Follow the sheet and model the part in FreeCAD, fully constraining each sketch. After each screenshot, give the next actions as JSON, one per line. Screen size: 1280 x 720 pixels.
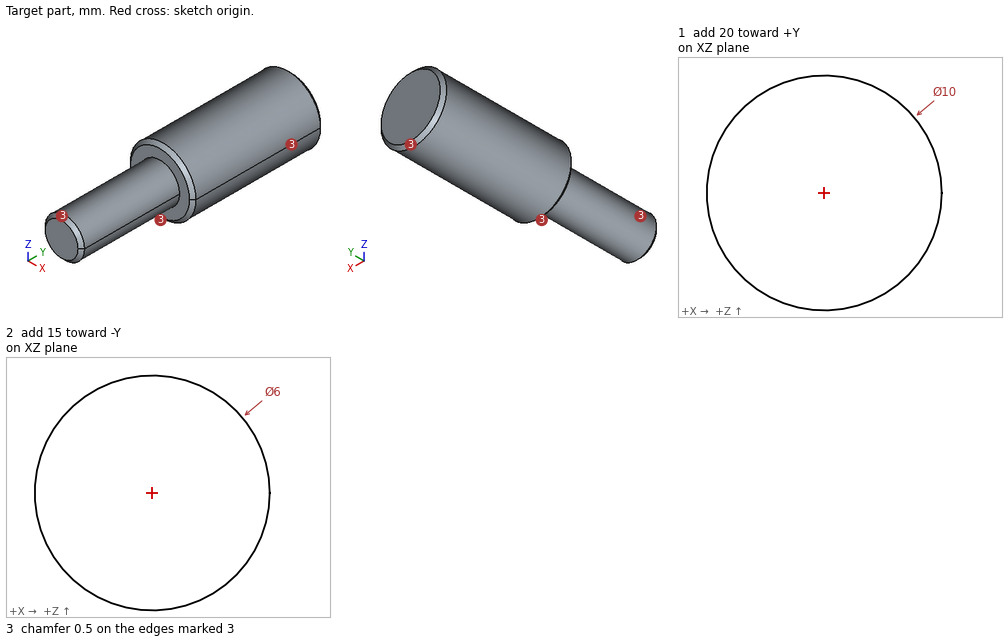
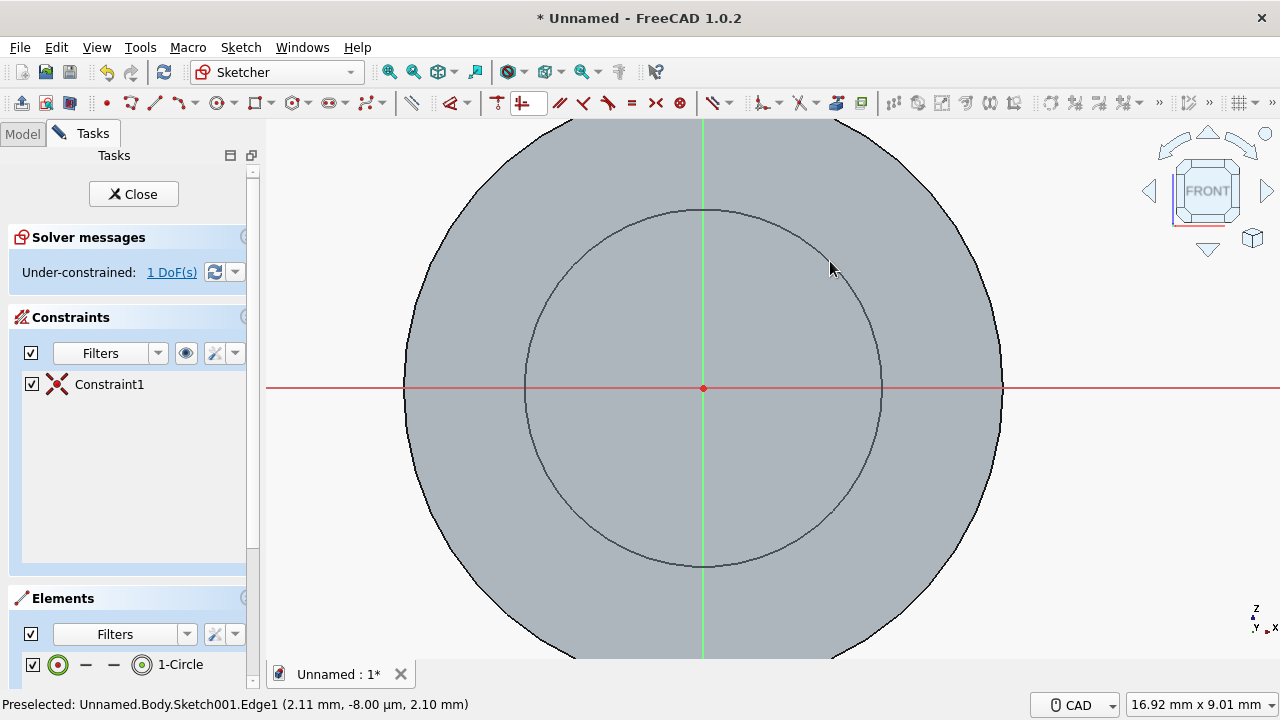
{"action": "left_click", "coordinate": [450, 104]}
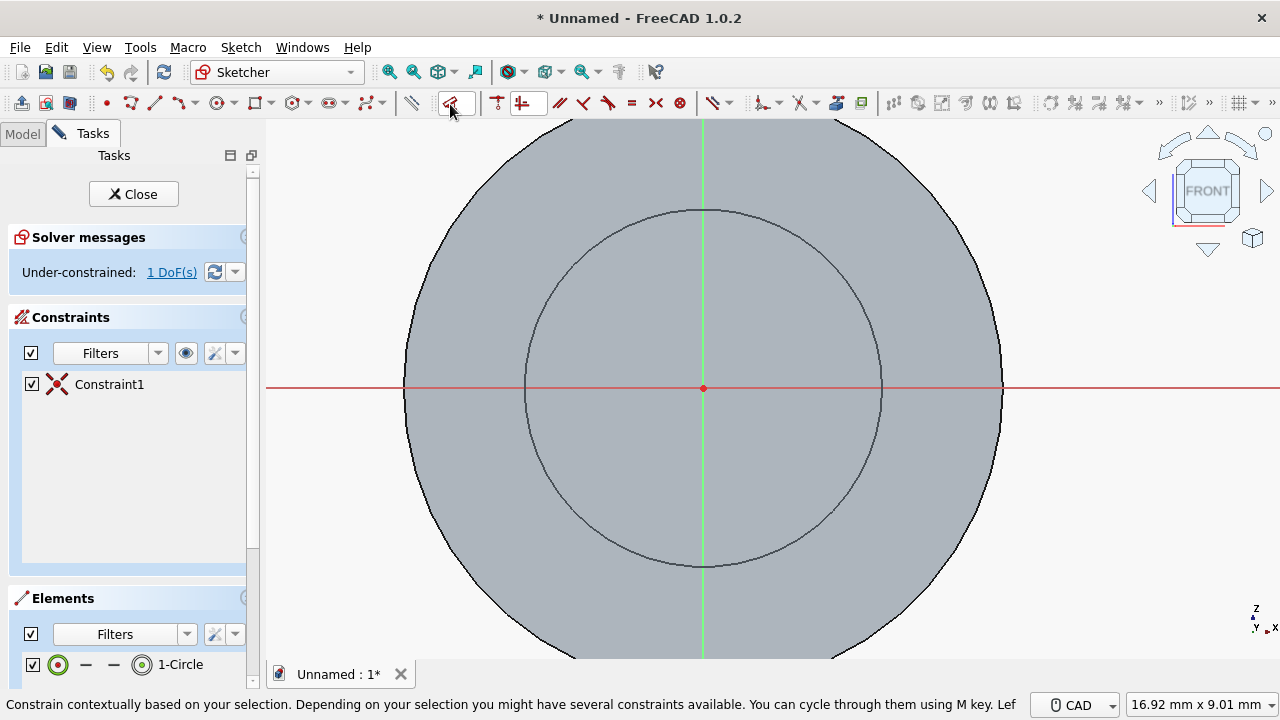
{"action": "left_click", "coordinate": [829, 261]}
{"action": "left_click", "coordinate": [851, 238]}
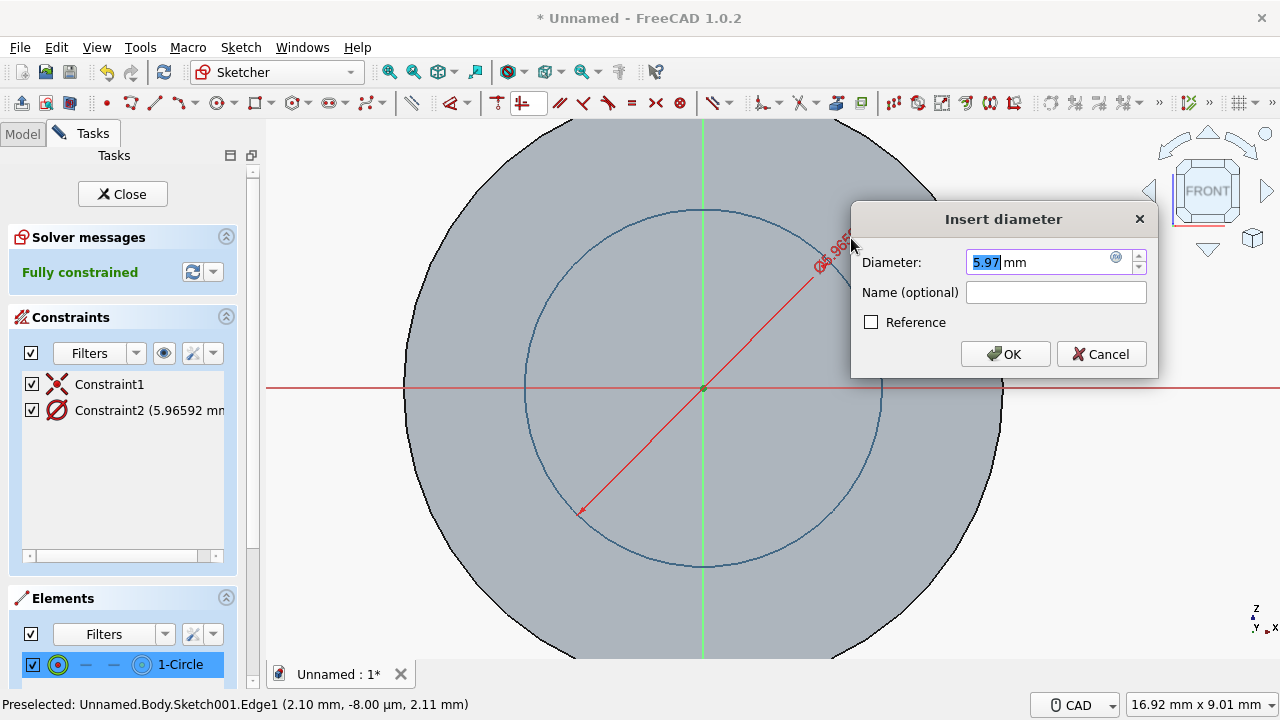
{"action": "type", "text": "6"}
{"action": "key", "text": "Return"}
{"action": "key", "text": "Escape"}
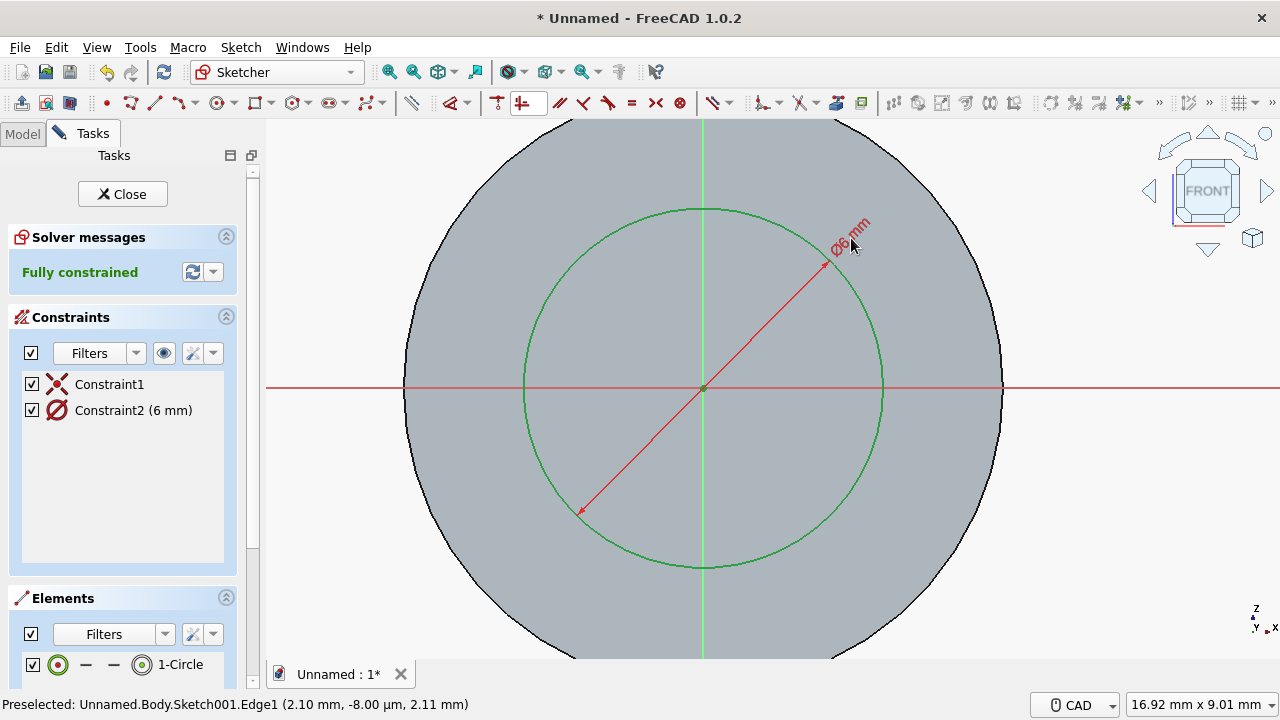
{"action": "left_click", "coordinate": [123, 194]}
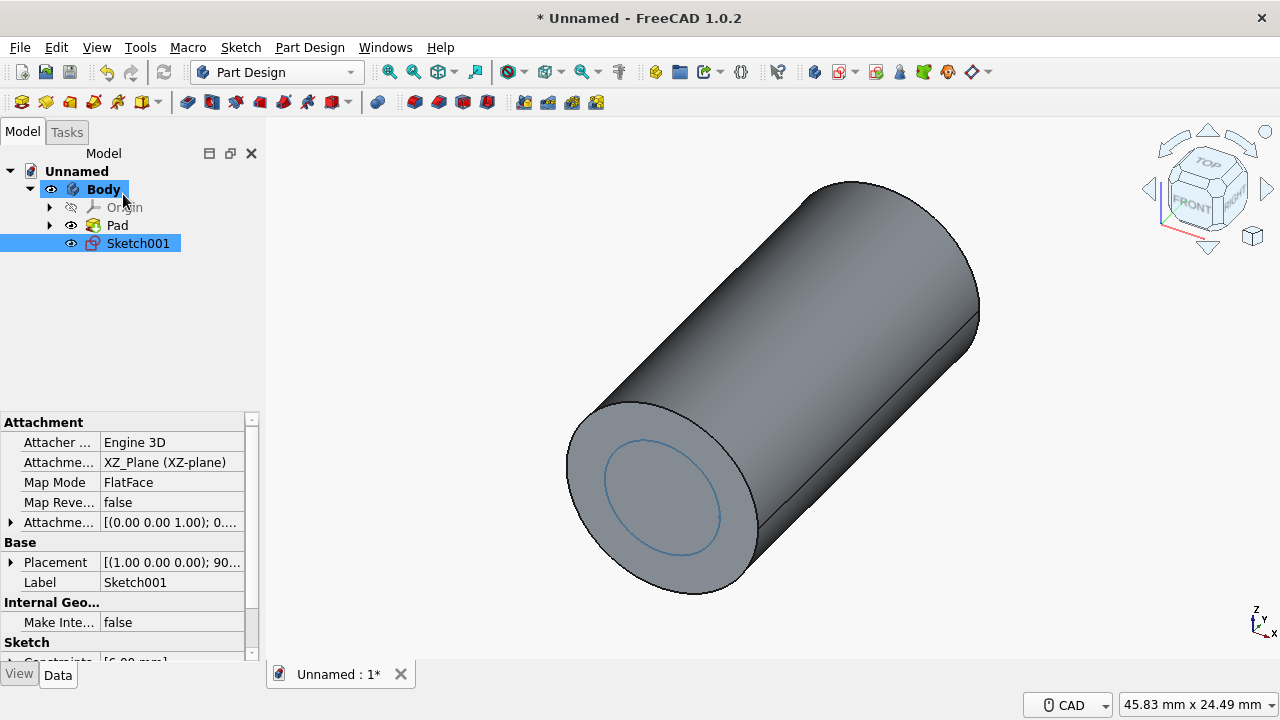
{"action": "left_click", "coordinate": [22, 102]}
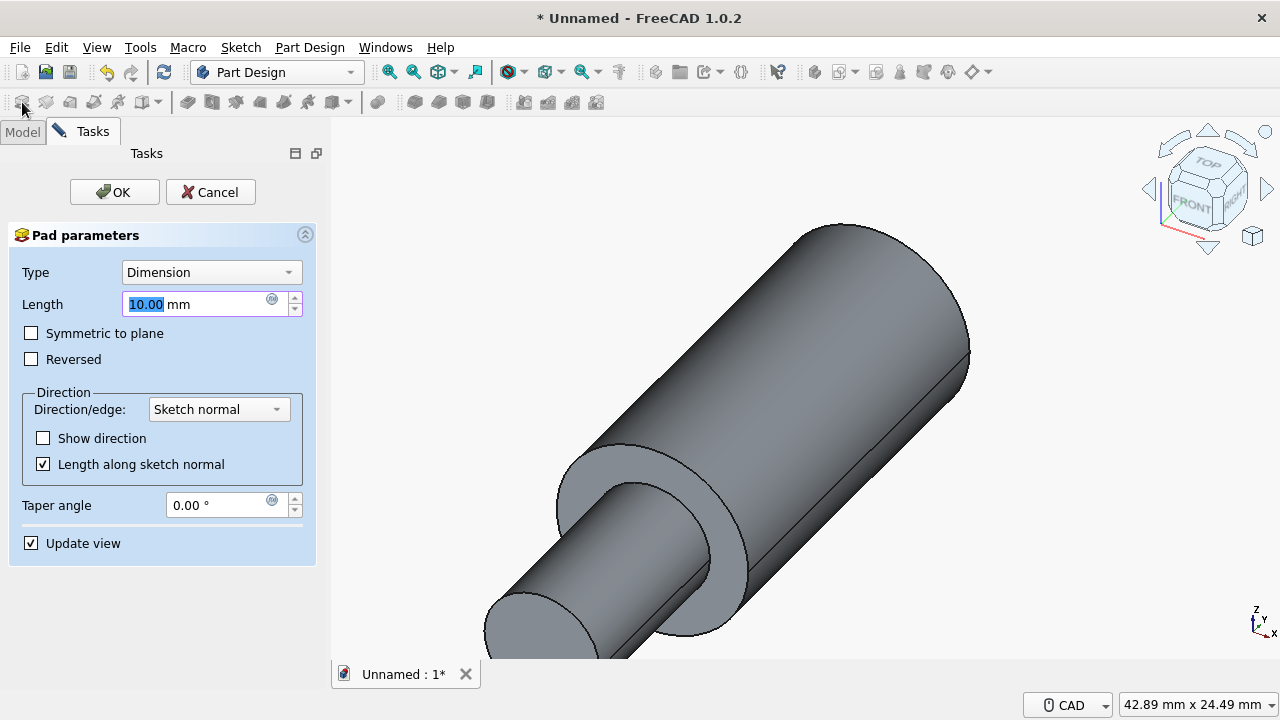
{"action": "type", "text": "15"}
{"action": "key", "text": "Tab"}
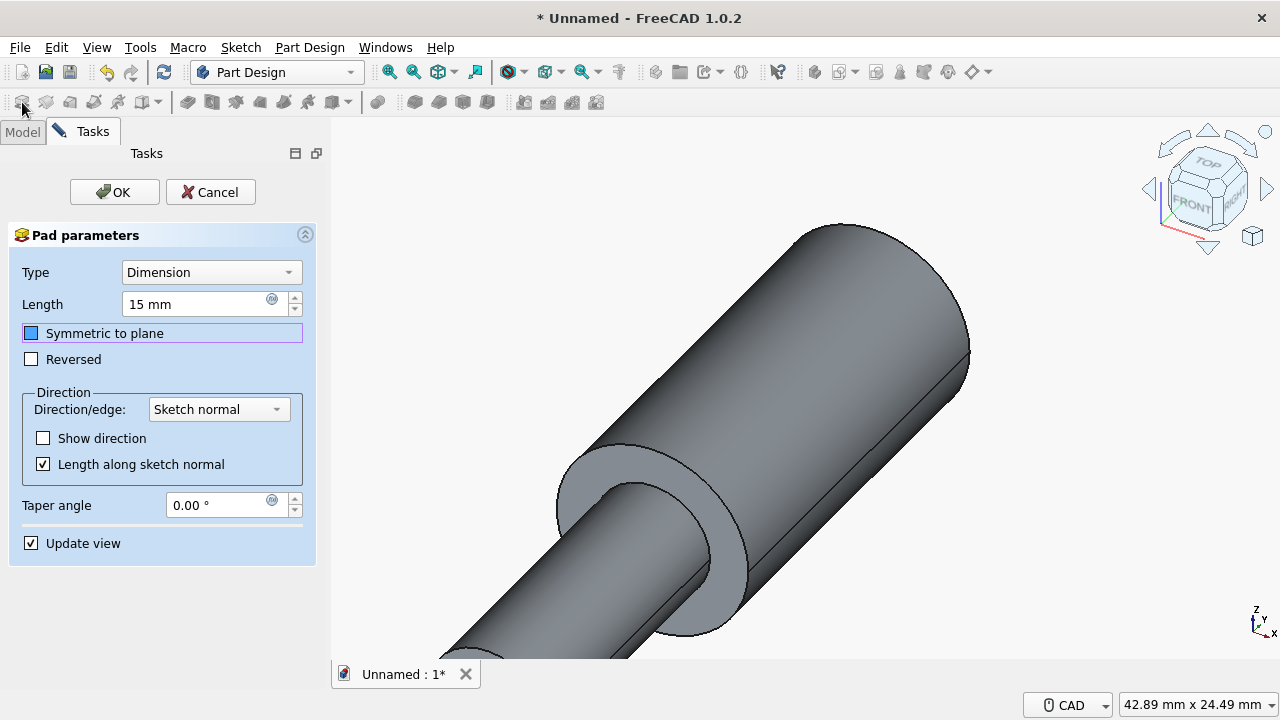
{"action": "left_click", "coordinate": [115, 192]}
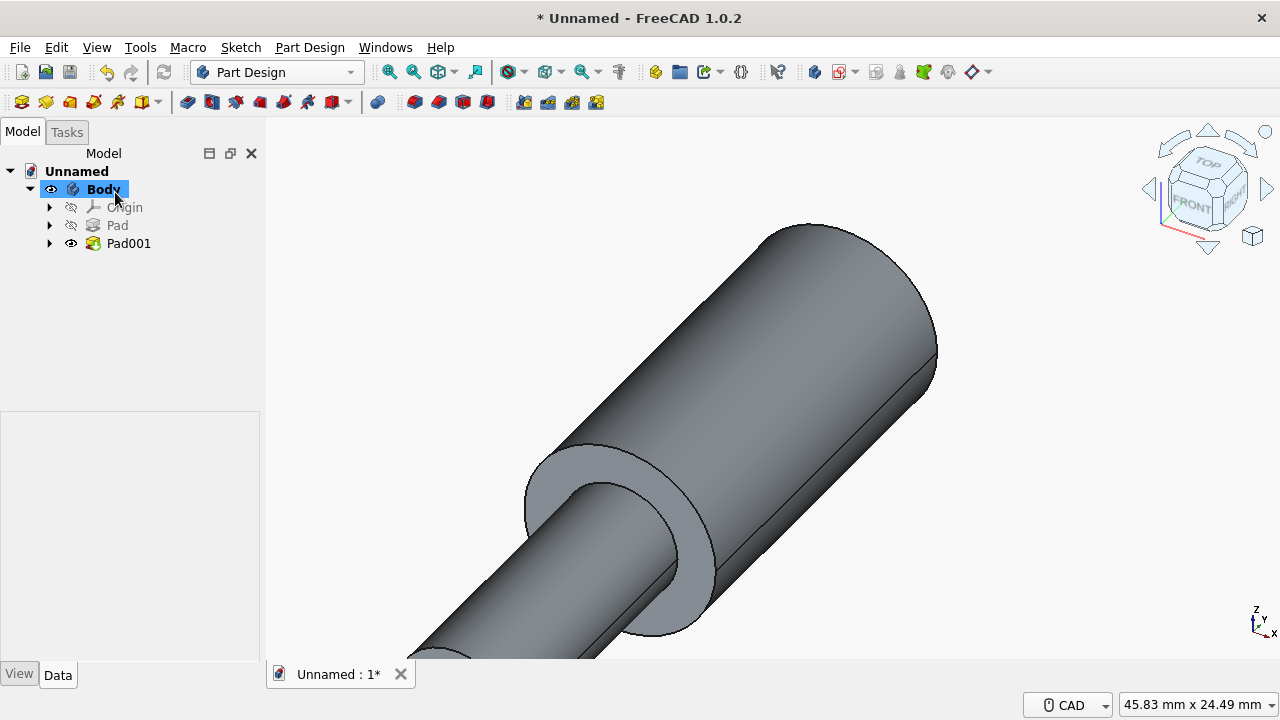
{"action": "left_click", "coordinate": [390, 72]}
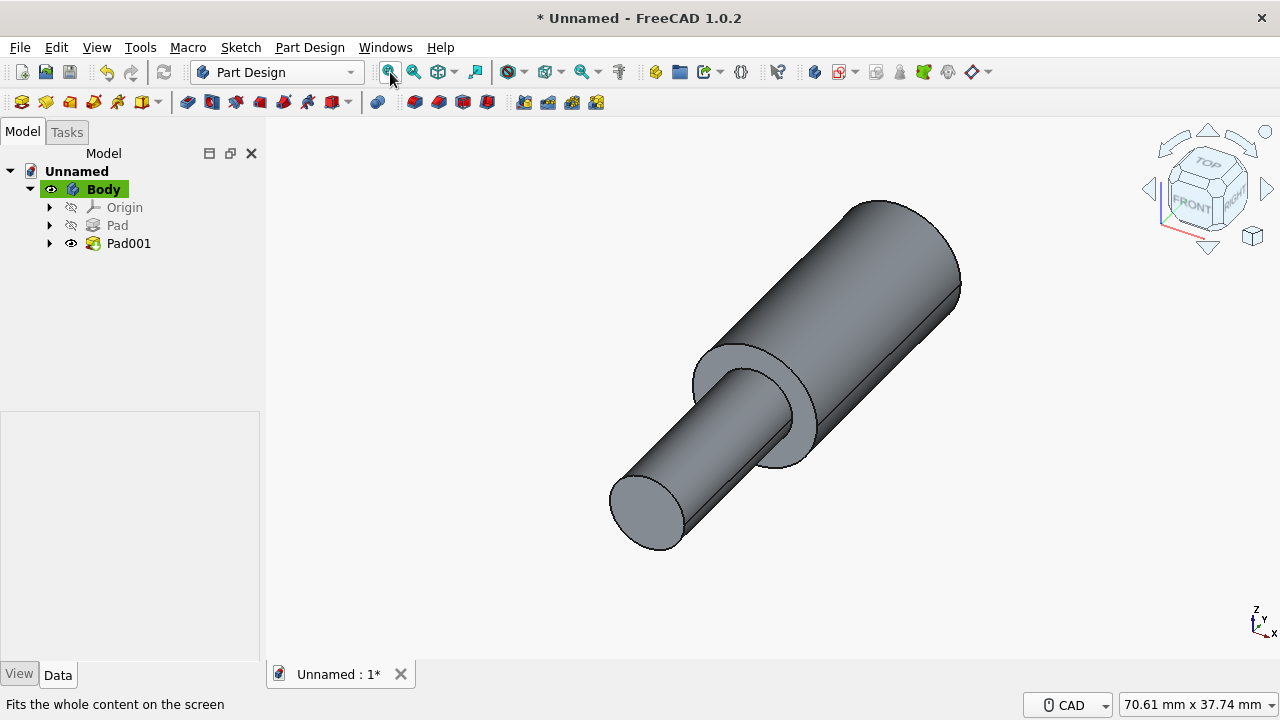
{"action": "left_click", "coordinate": [705, 354]}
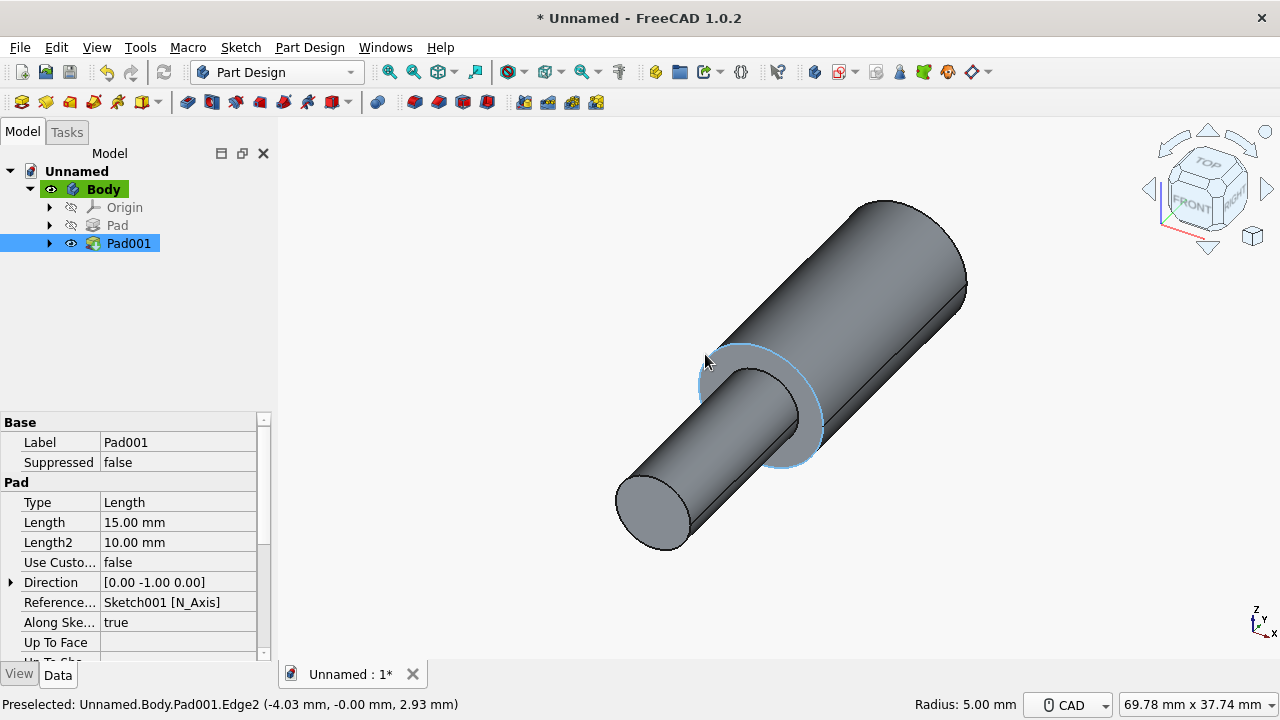
{"action": "left_click", "coordinate": [623, 481], "text": "ctrl"}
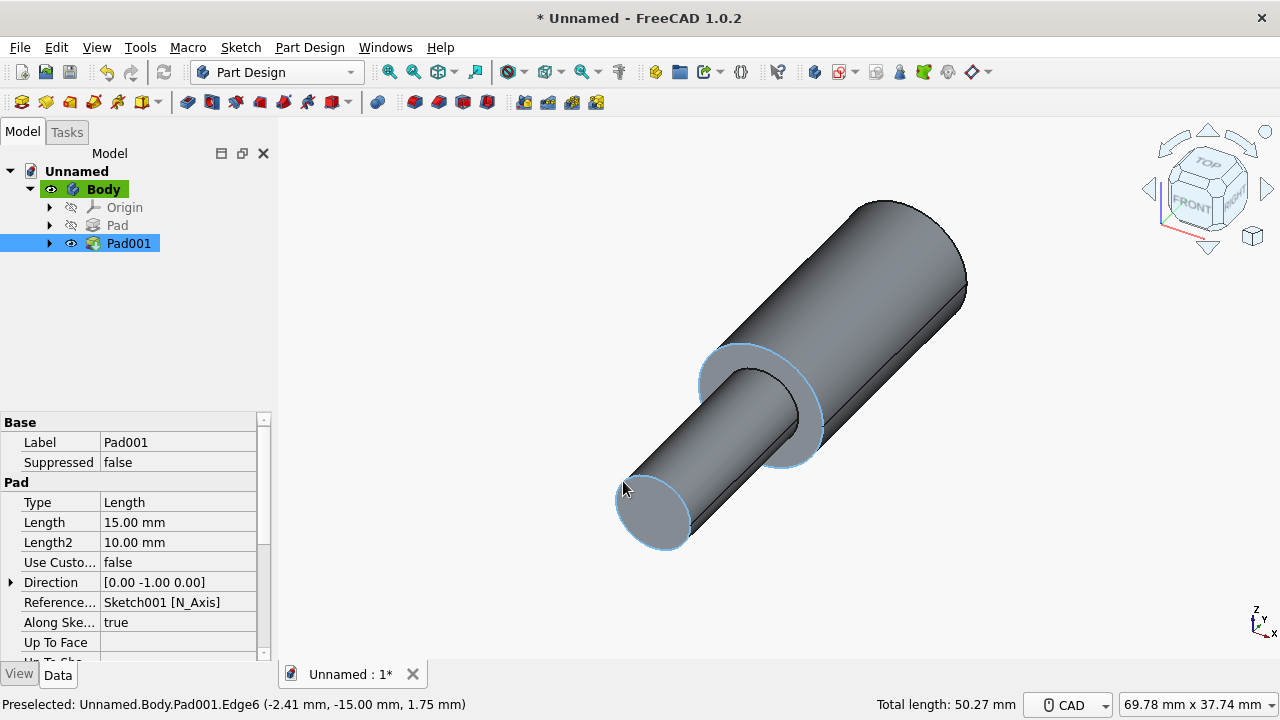
{"action": "key", "text": "0"}